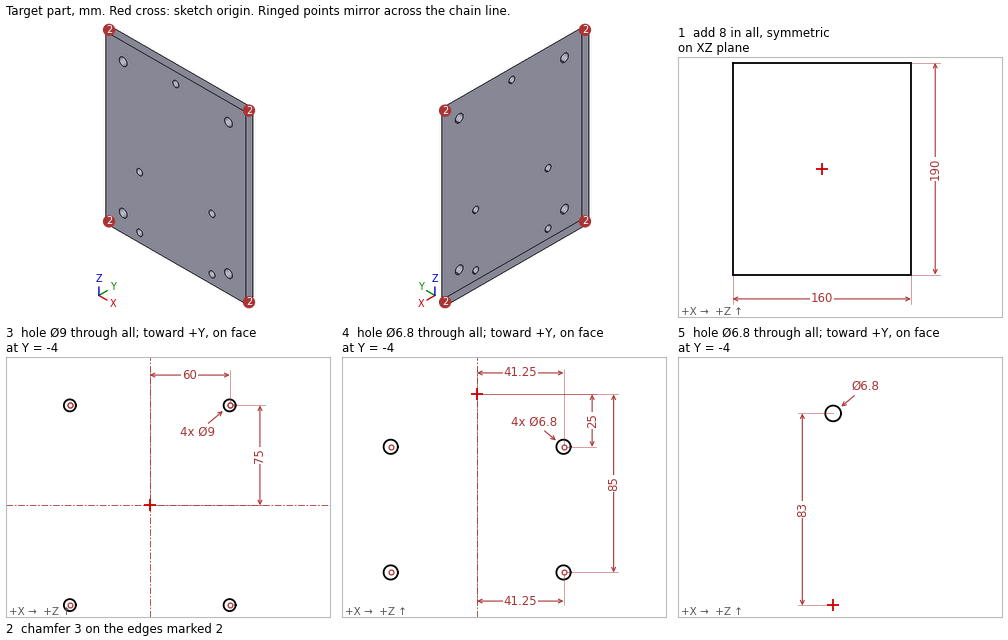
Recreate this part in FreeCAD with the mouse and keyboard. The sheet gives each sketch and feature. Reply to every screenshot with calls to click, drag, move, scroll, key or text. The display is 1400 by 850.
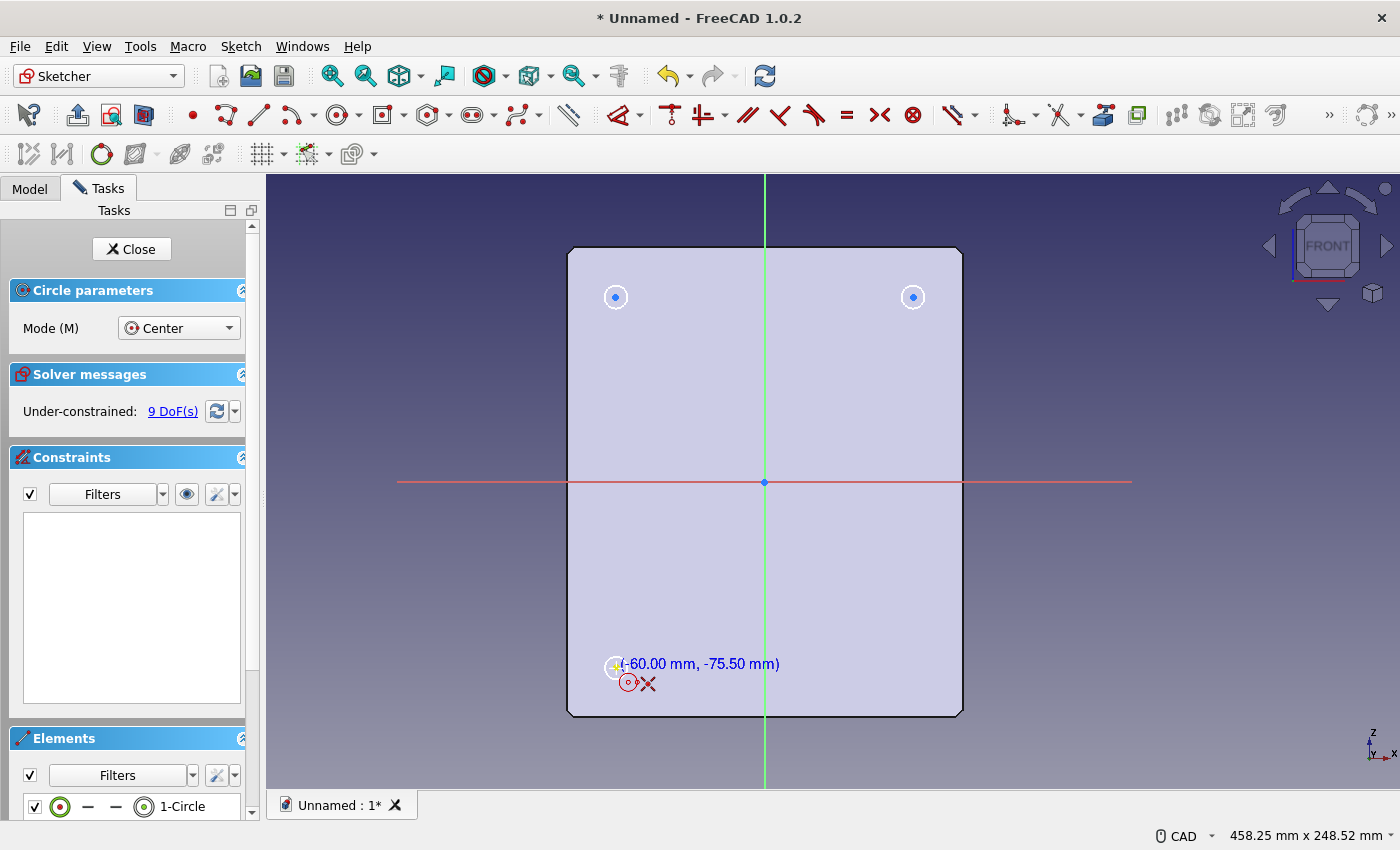
scroll(913, 668, up, 4)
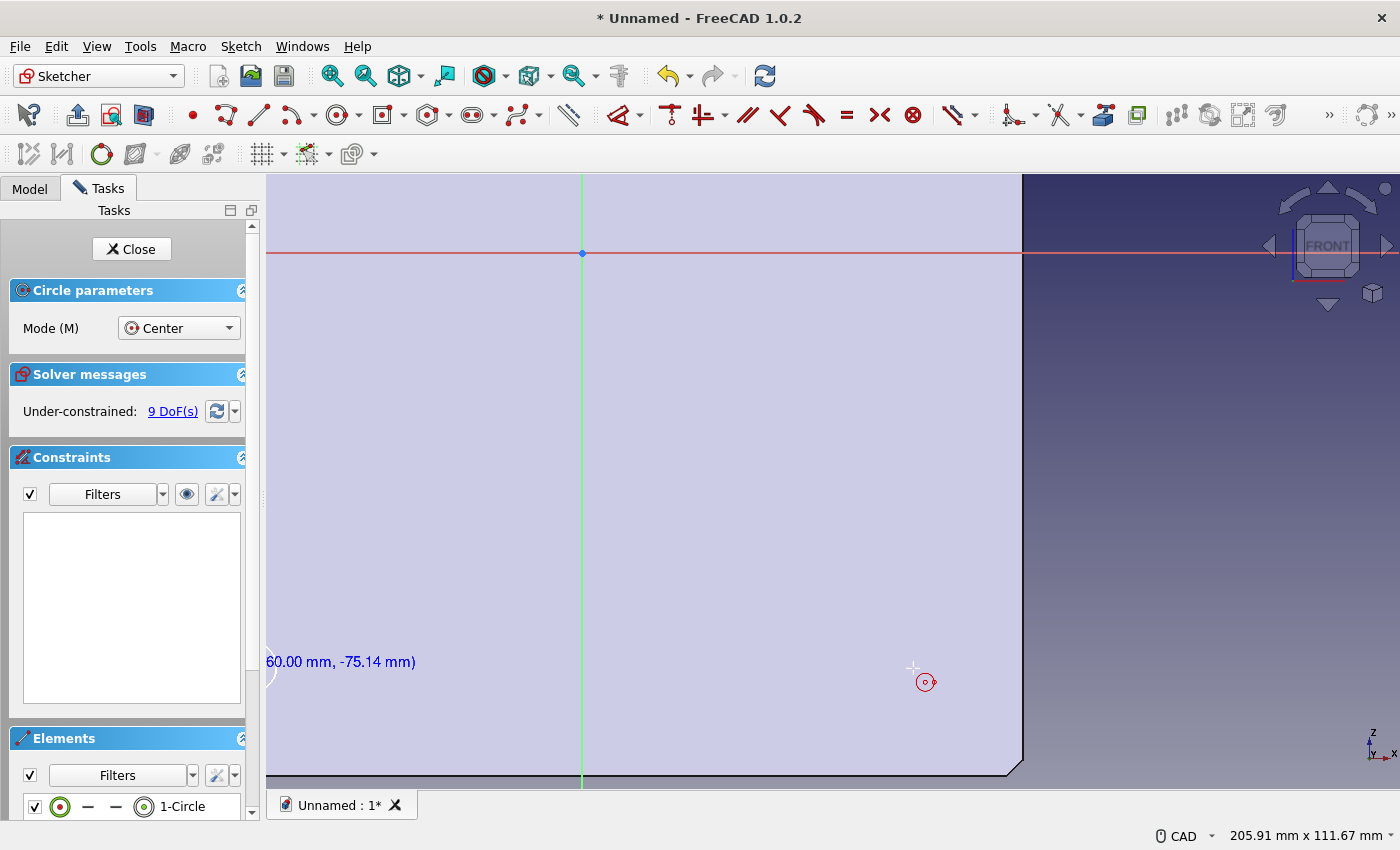
click(913, 666)
click(930, 649)
key(Escape)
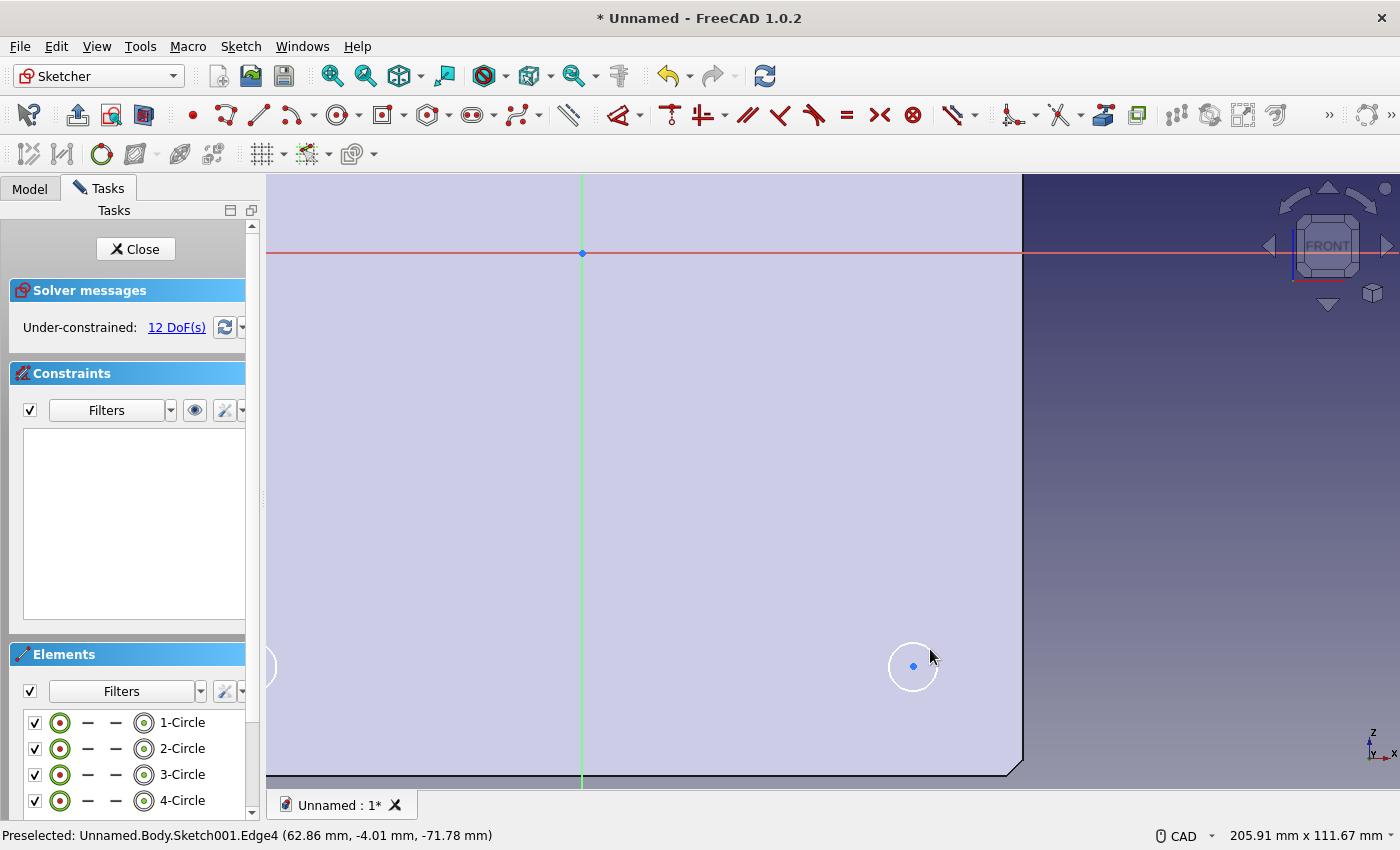
scroll(913, 668, down, 4)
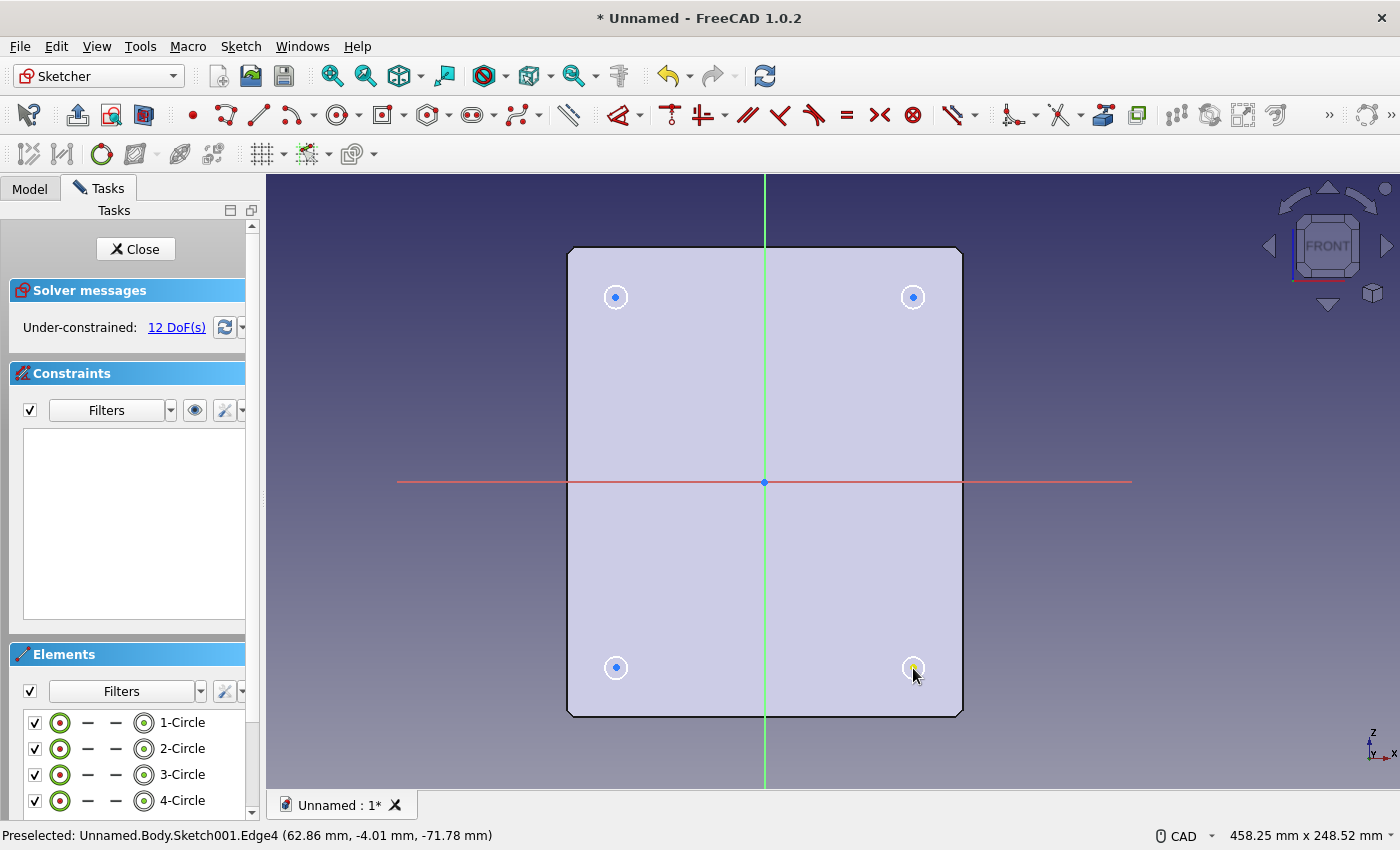
click(921, 289)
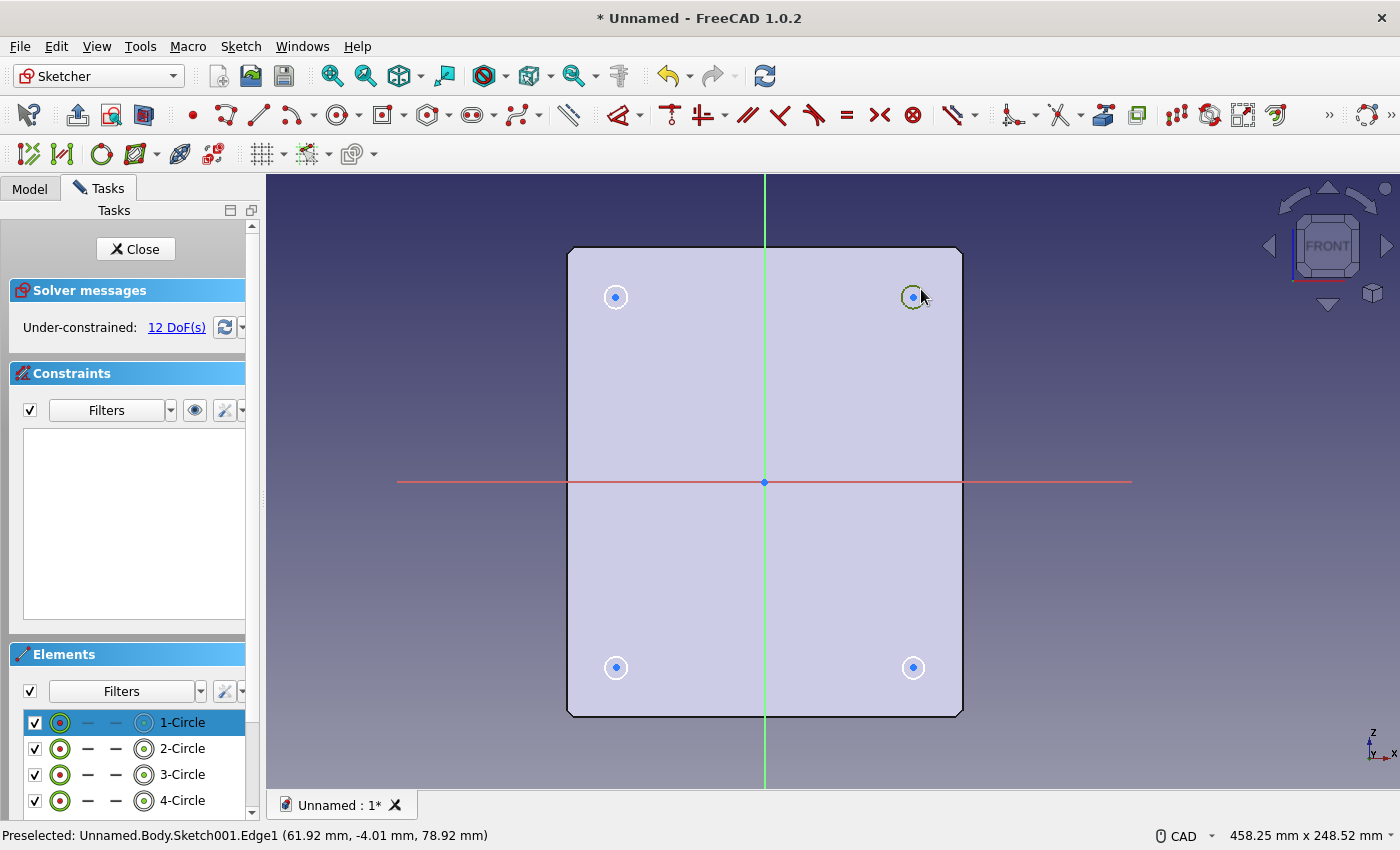
click(624, 289)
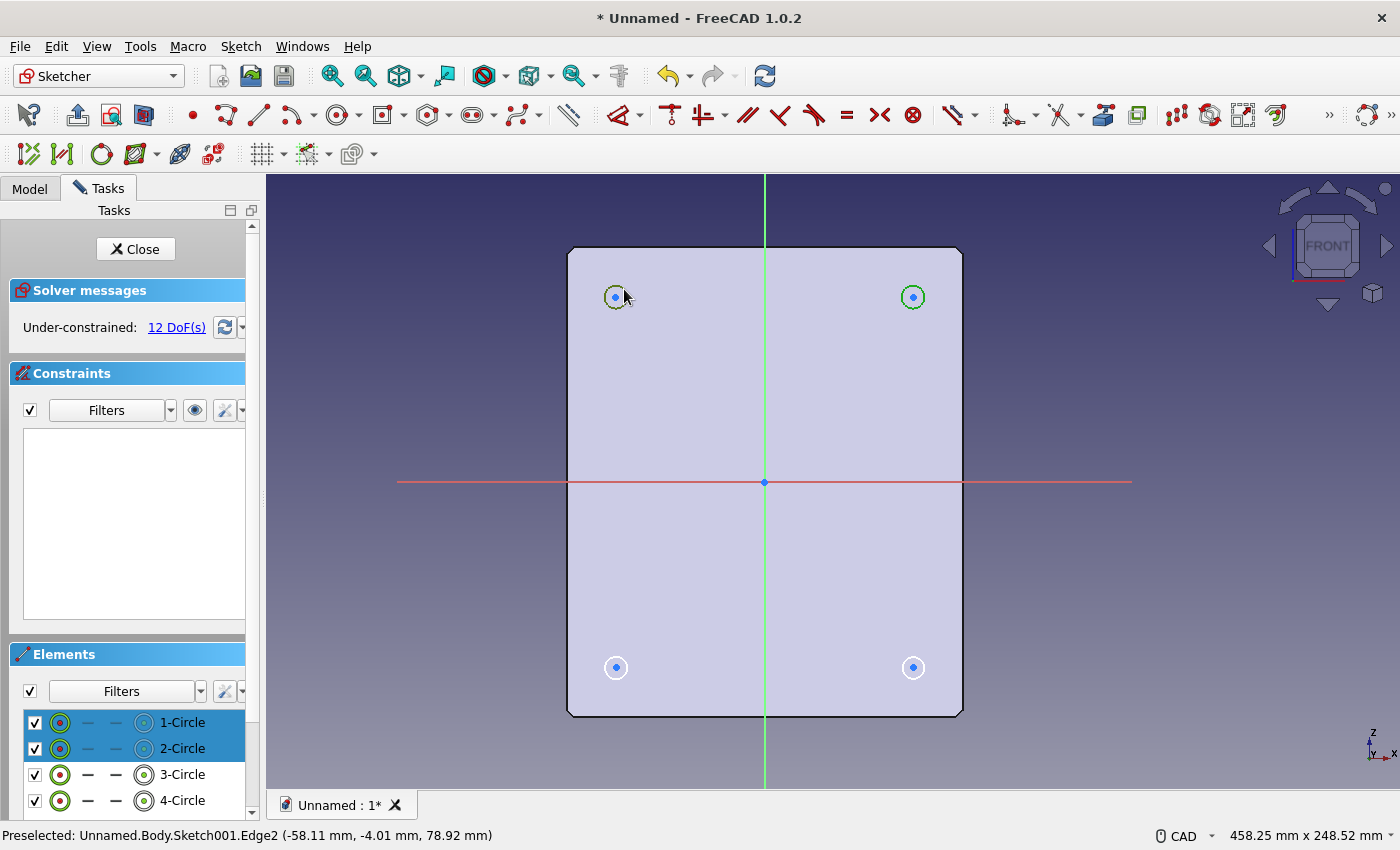
scroll(624, 660, up, 2)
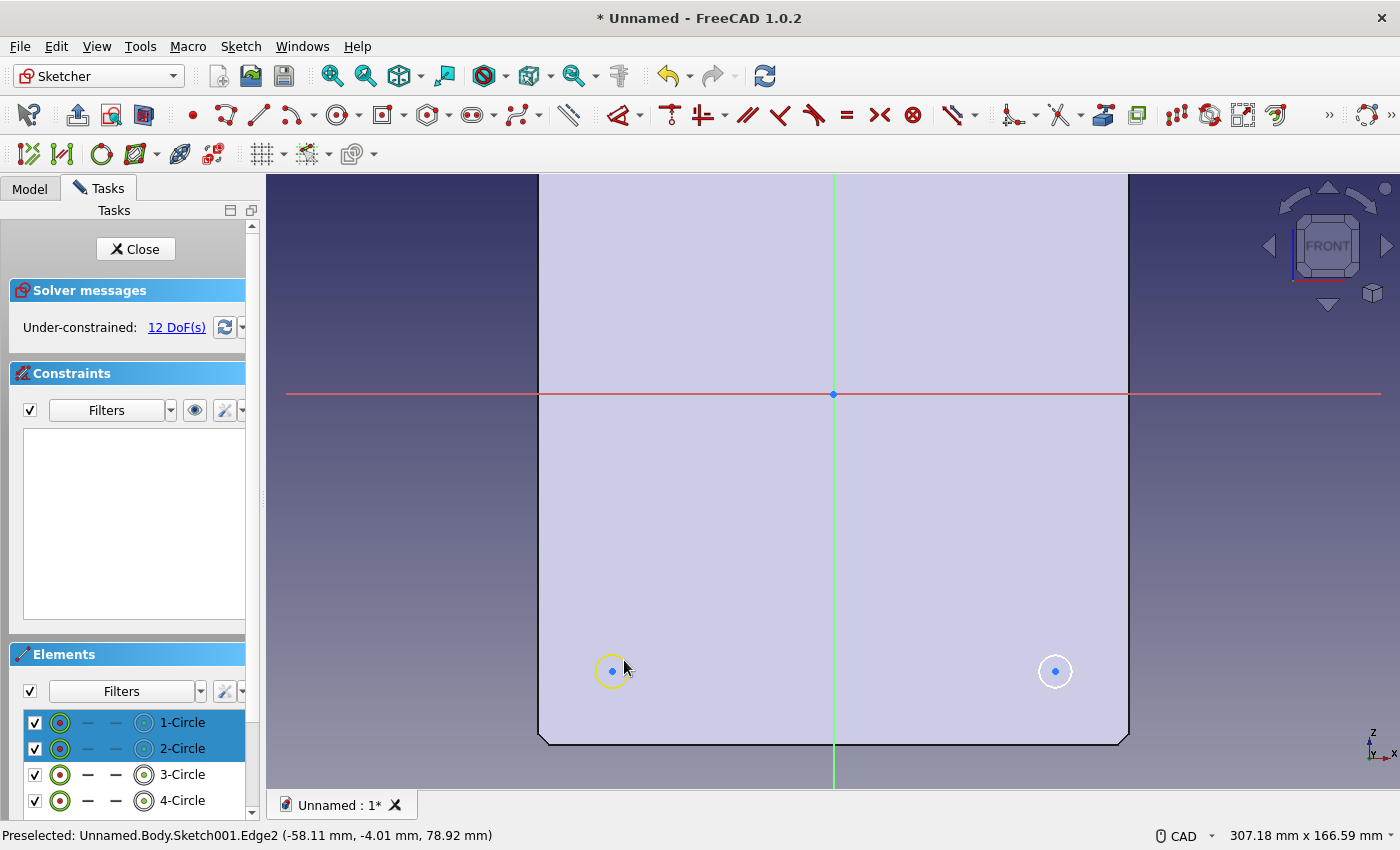
click(624, 660)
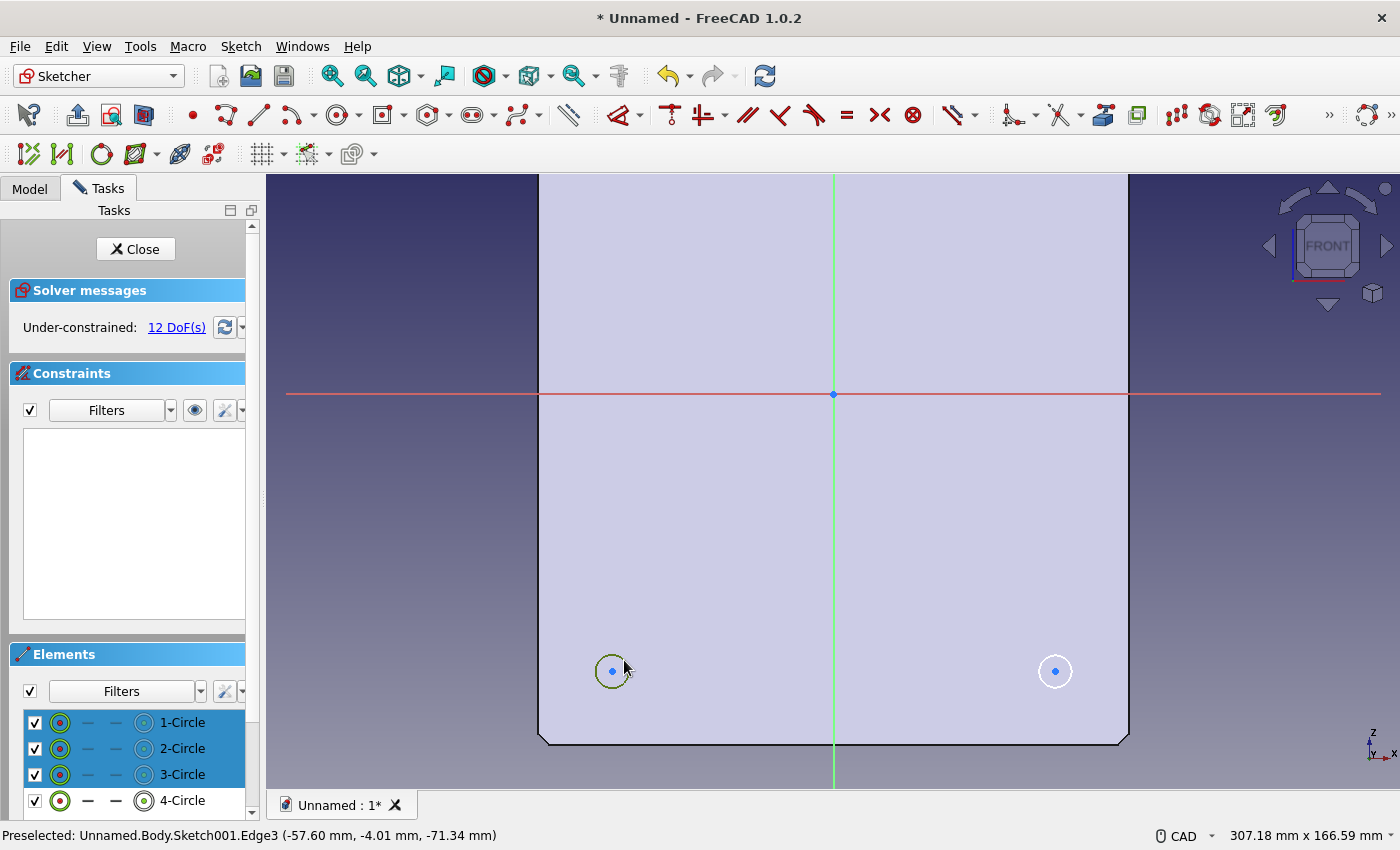
click(1067, 660)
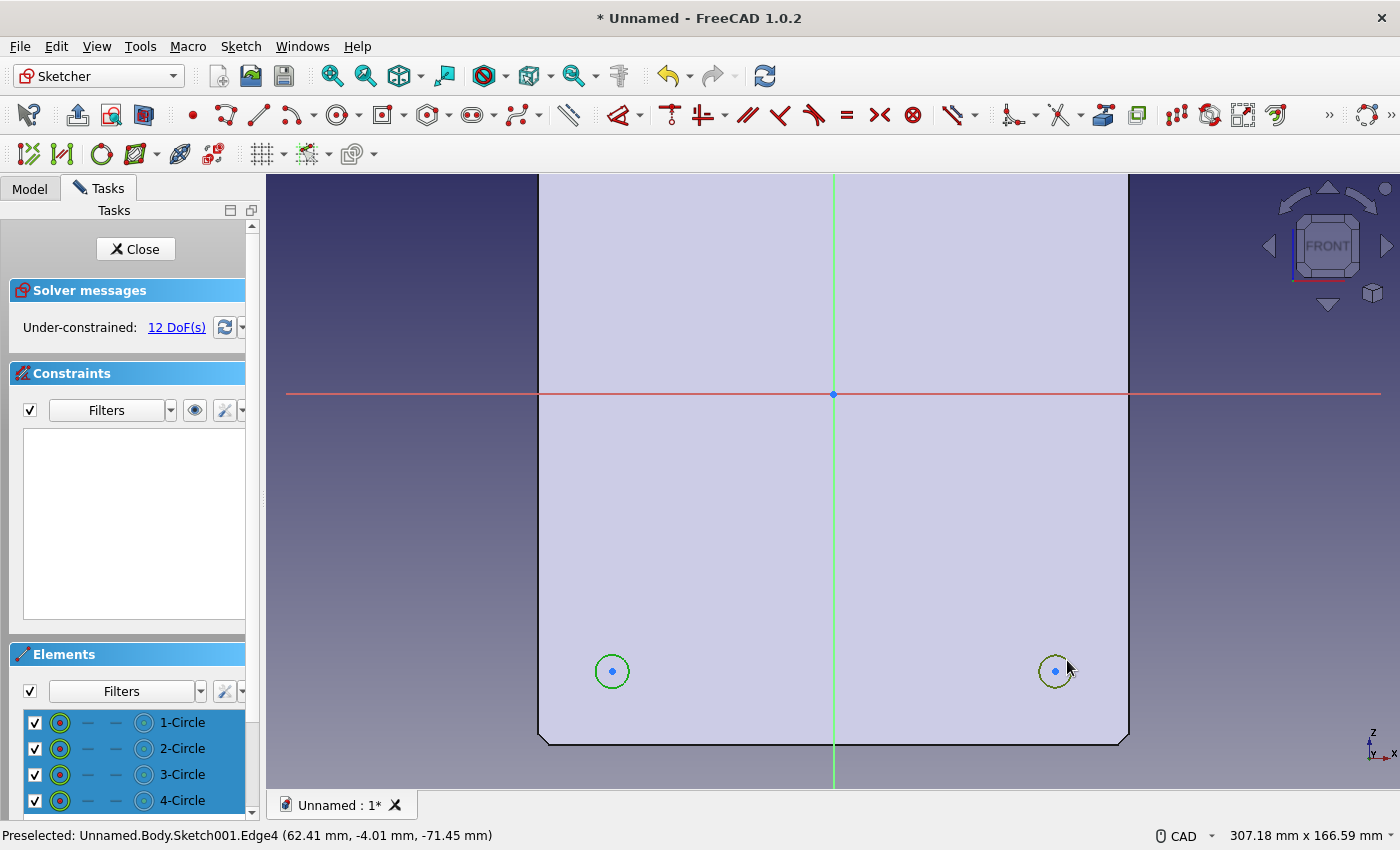
click(847, 116)